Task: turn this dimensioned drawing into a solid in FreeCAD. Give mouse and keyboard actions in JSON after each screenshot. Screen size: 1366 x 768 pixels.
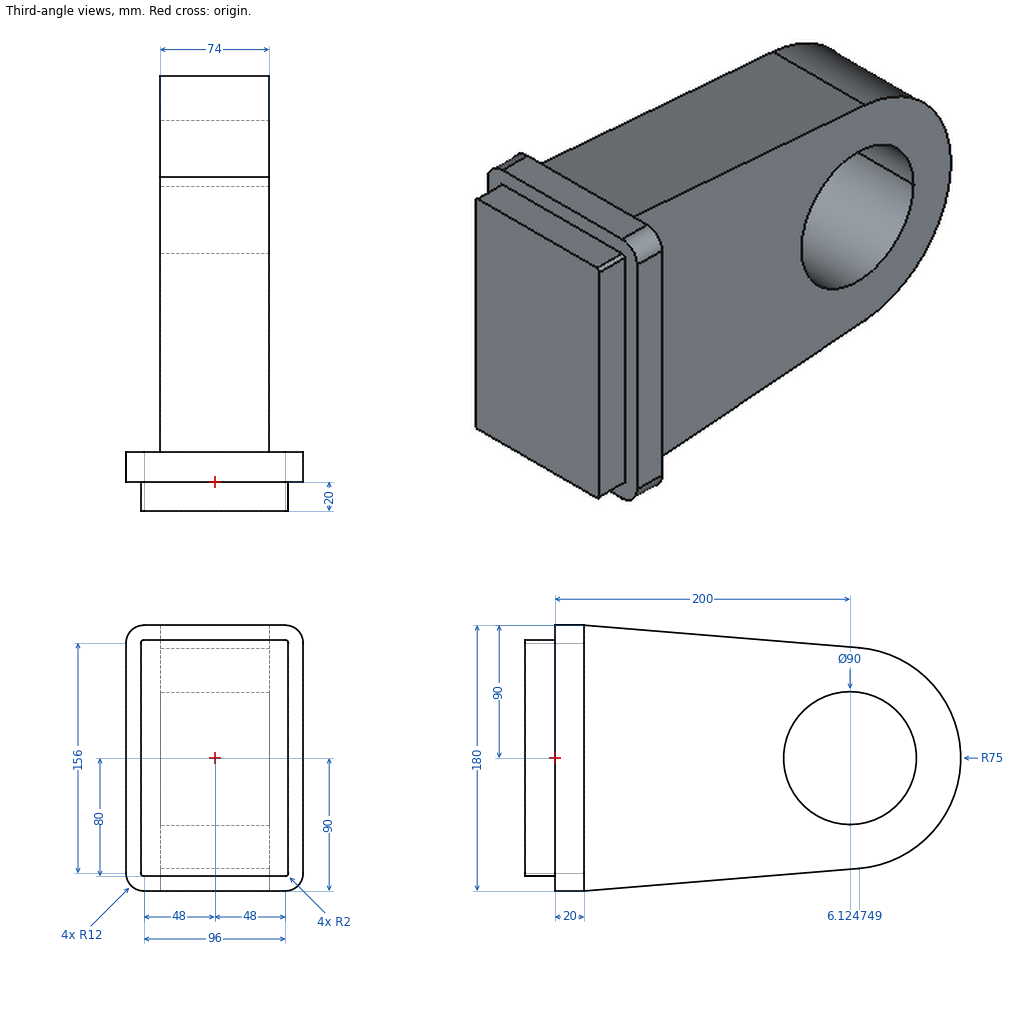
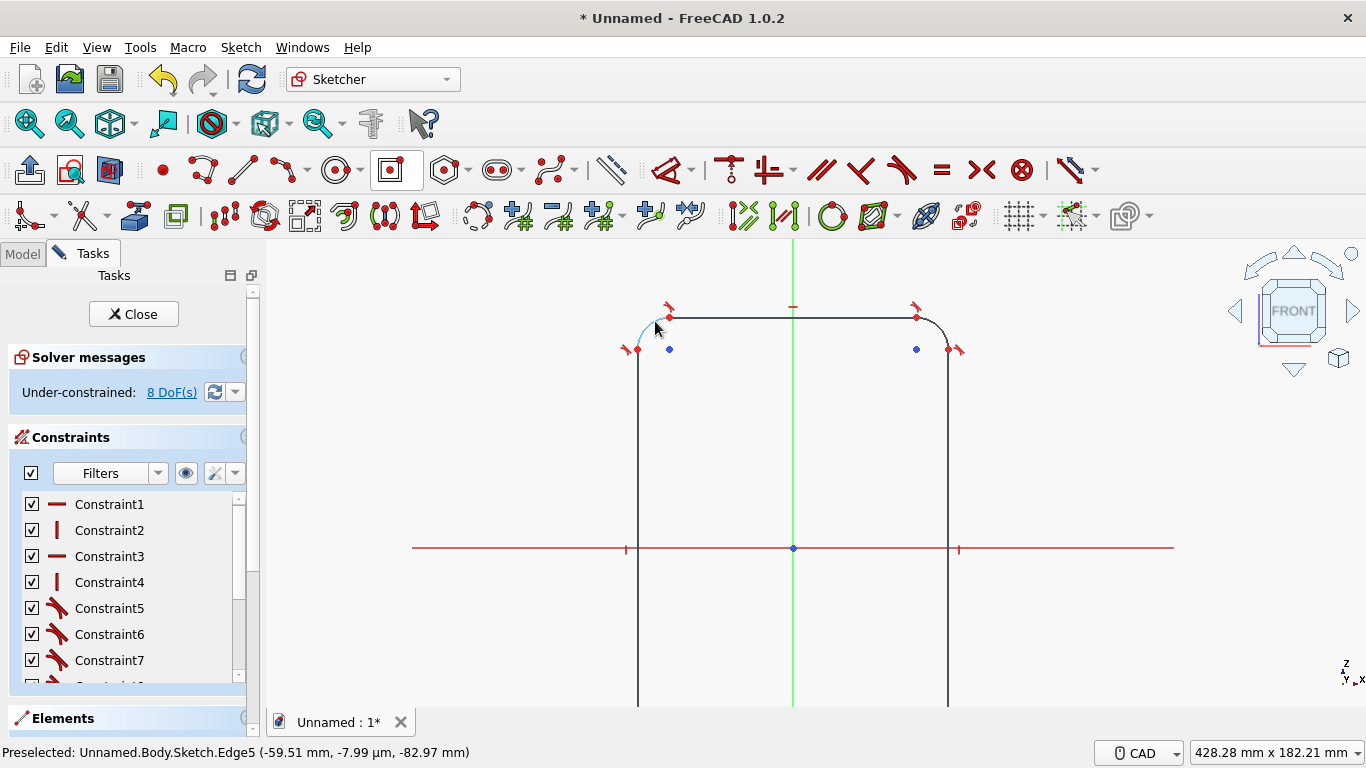
{"action": "left_click", "coordinate": [655, 321]}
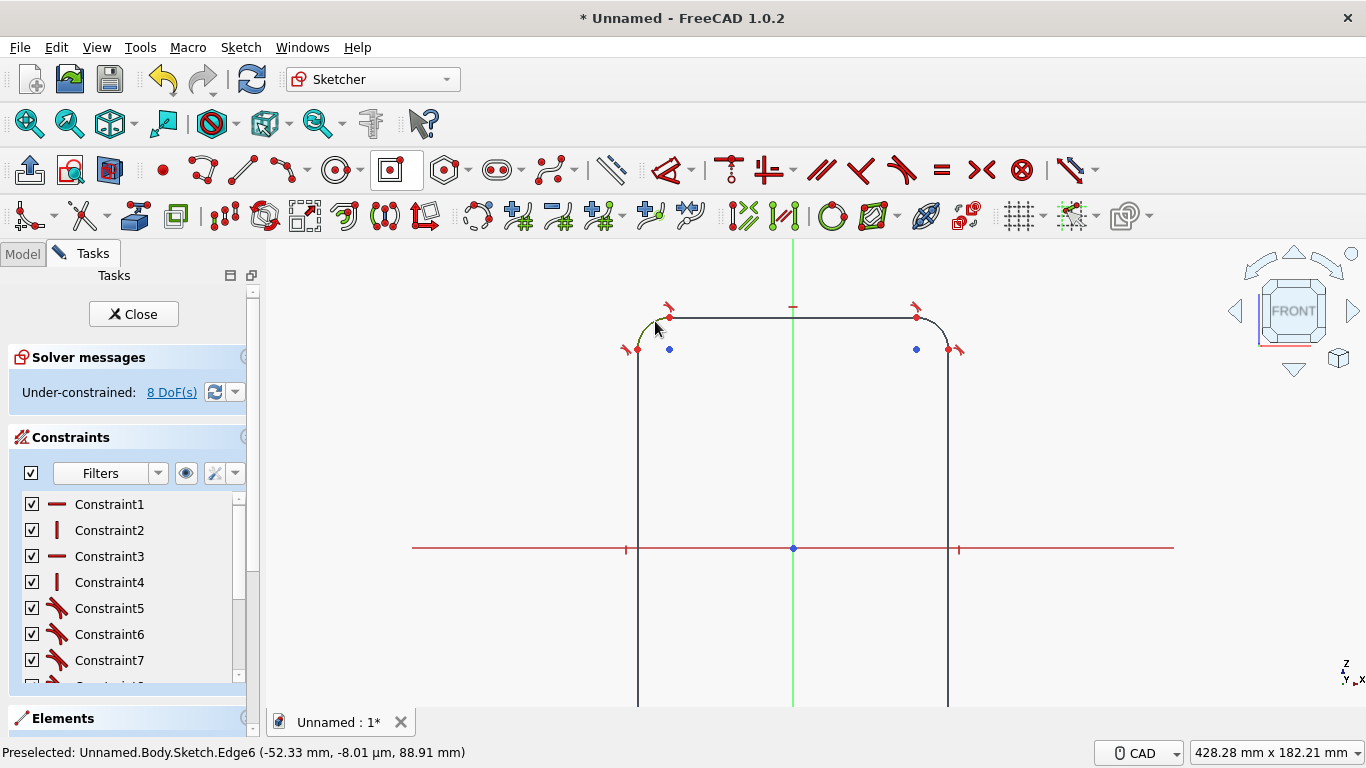
{"action": "left_click", "coordinate": [945, 335]}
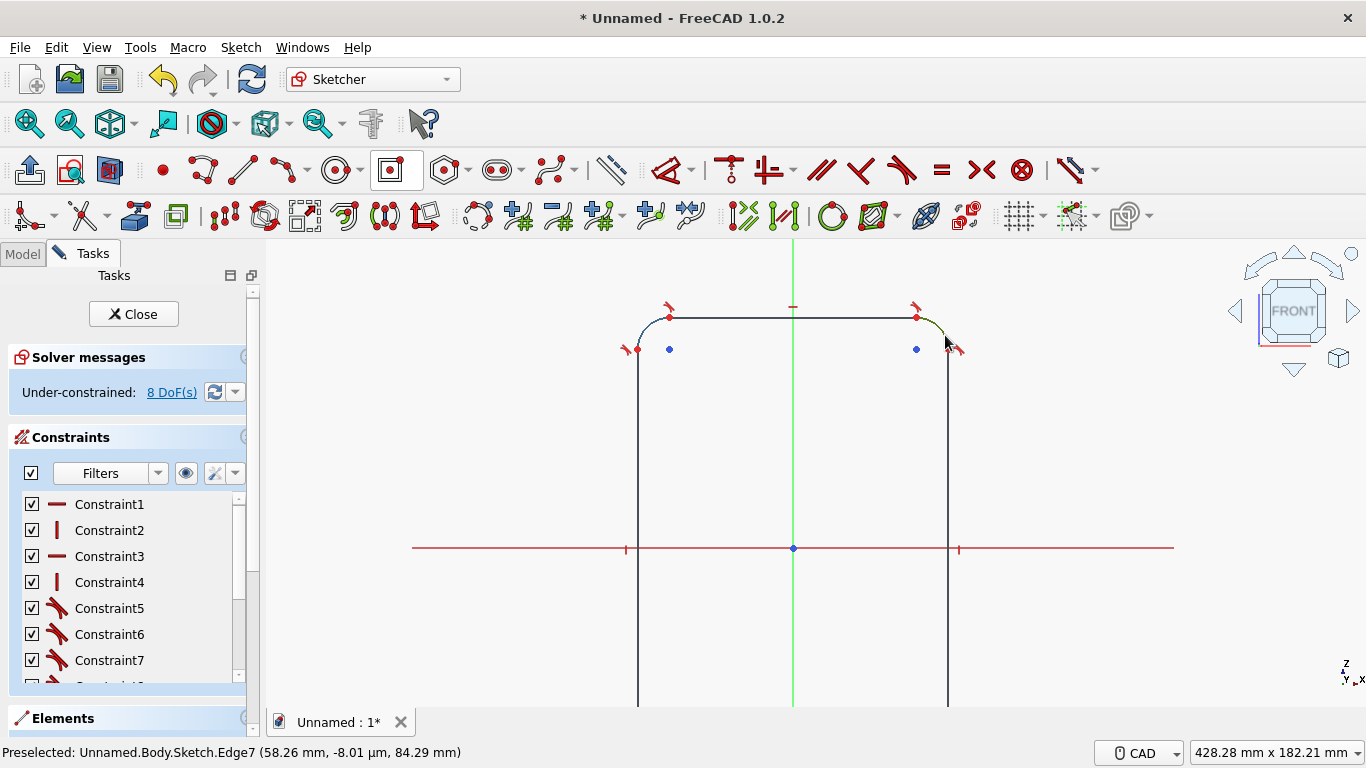
{"action": "scroll", "coordinate": [655, 320], "scroll_direction": "down", "scroll_amount": 2}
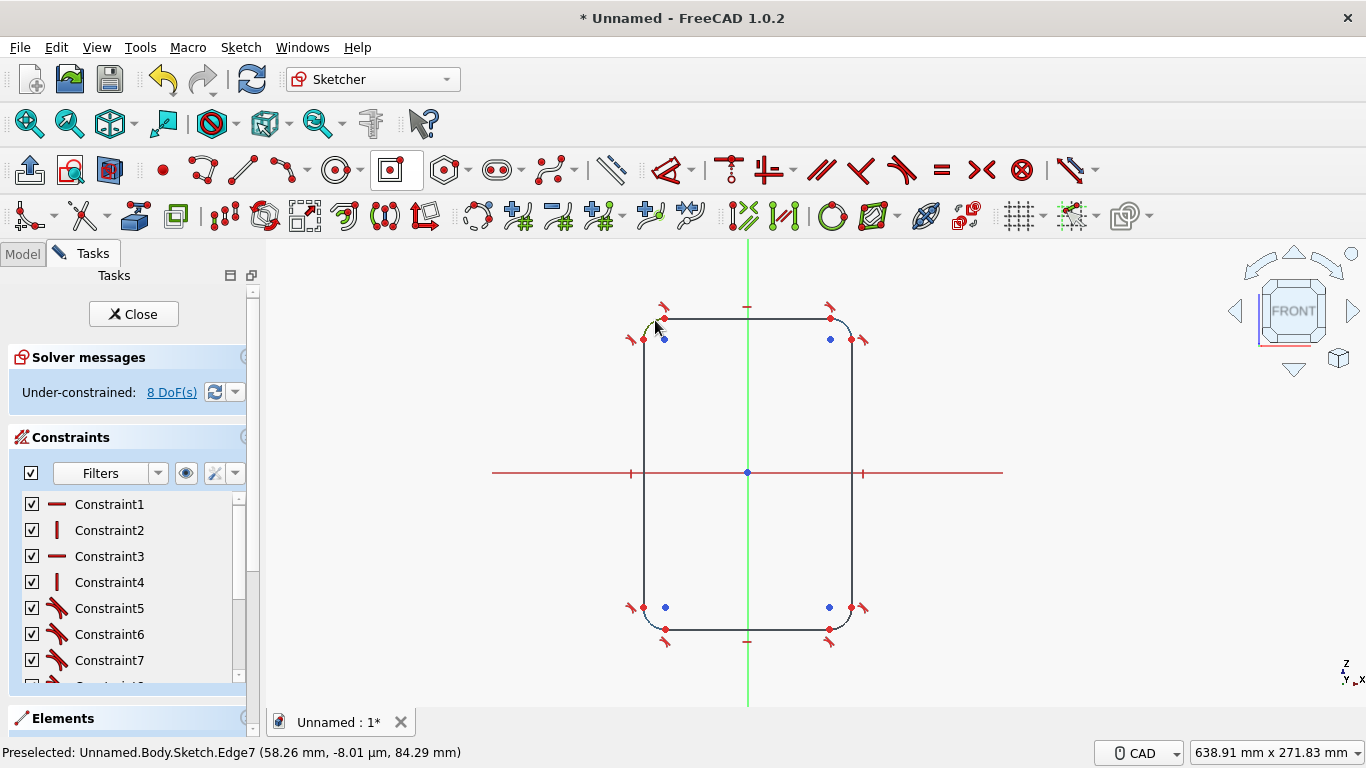
{"action": "scroll", "coordinate": [840, 627], "scroll_direction": "up", "scroll_amount": 2}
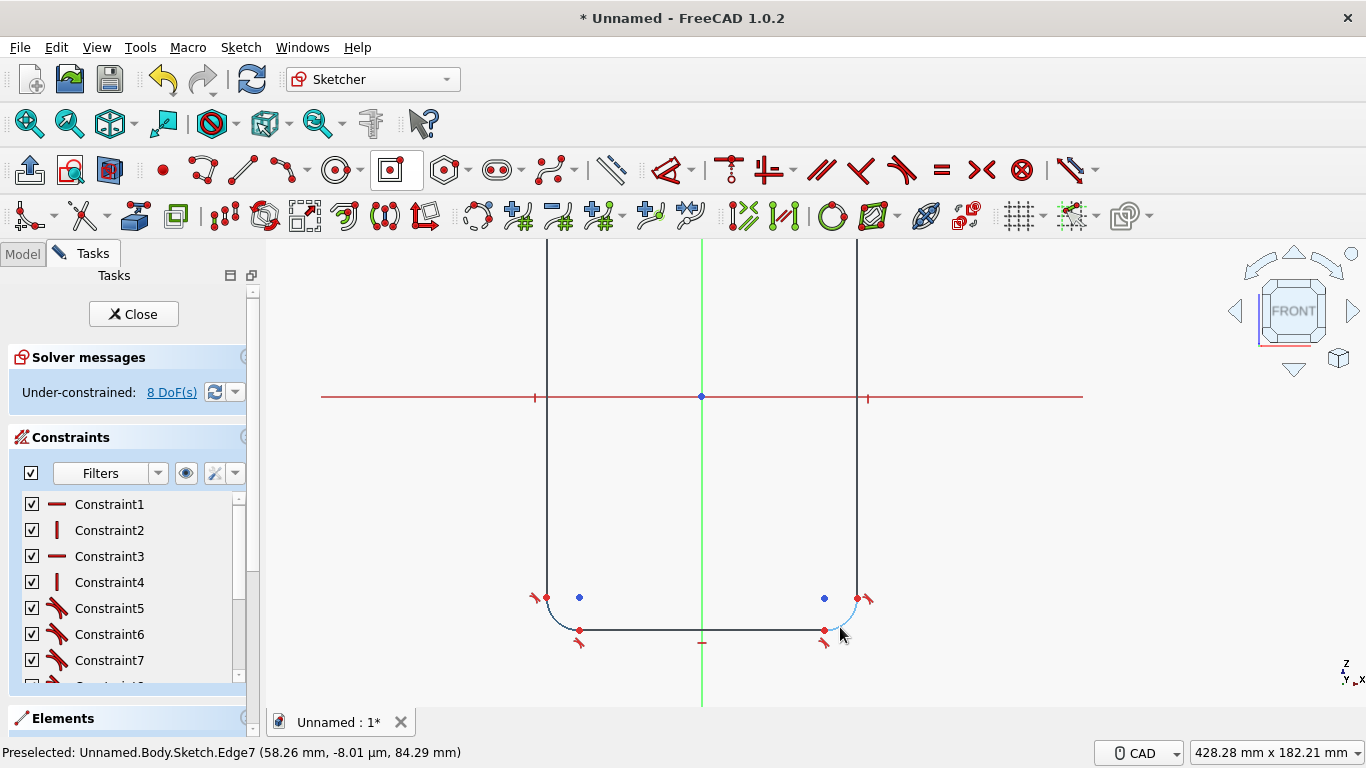
{"action": "left_click", "coordinate": [839, 627]}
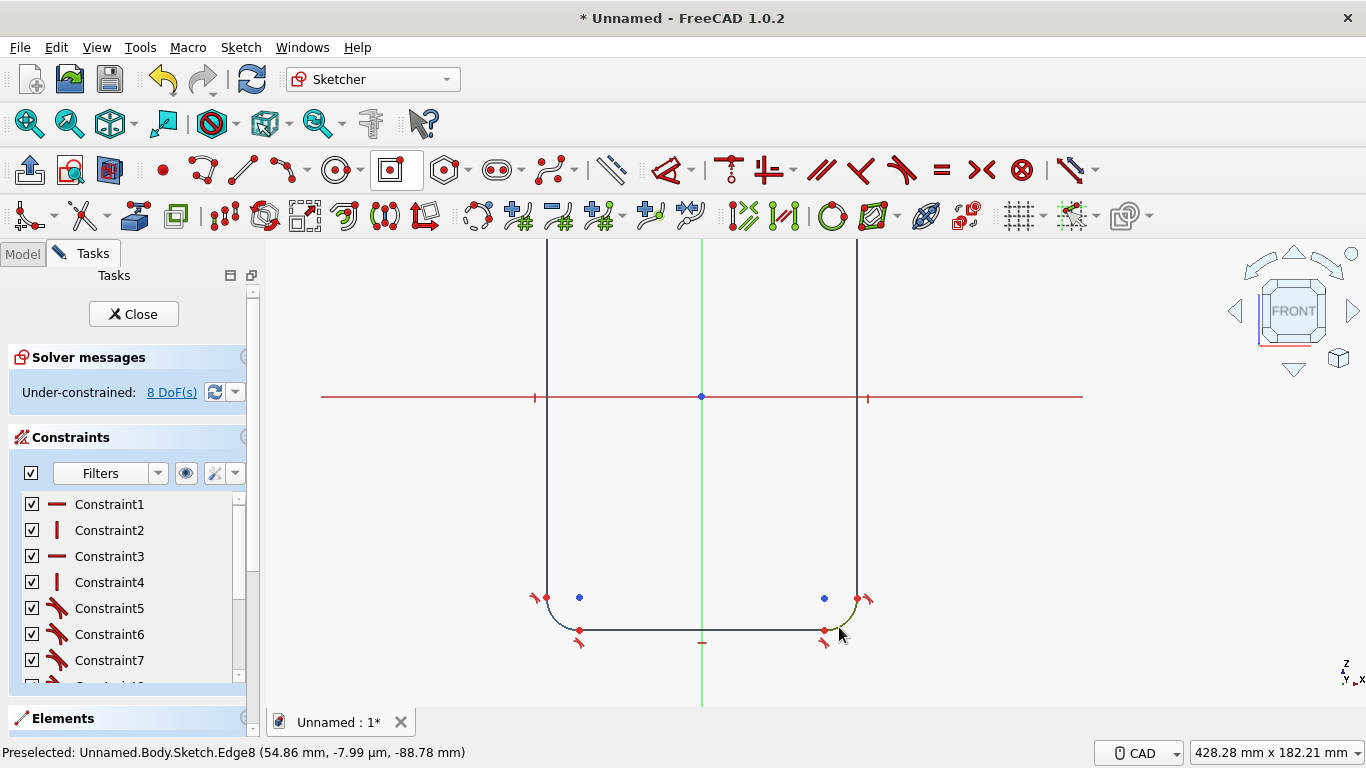
{"action": "key", "text": "e"}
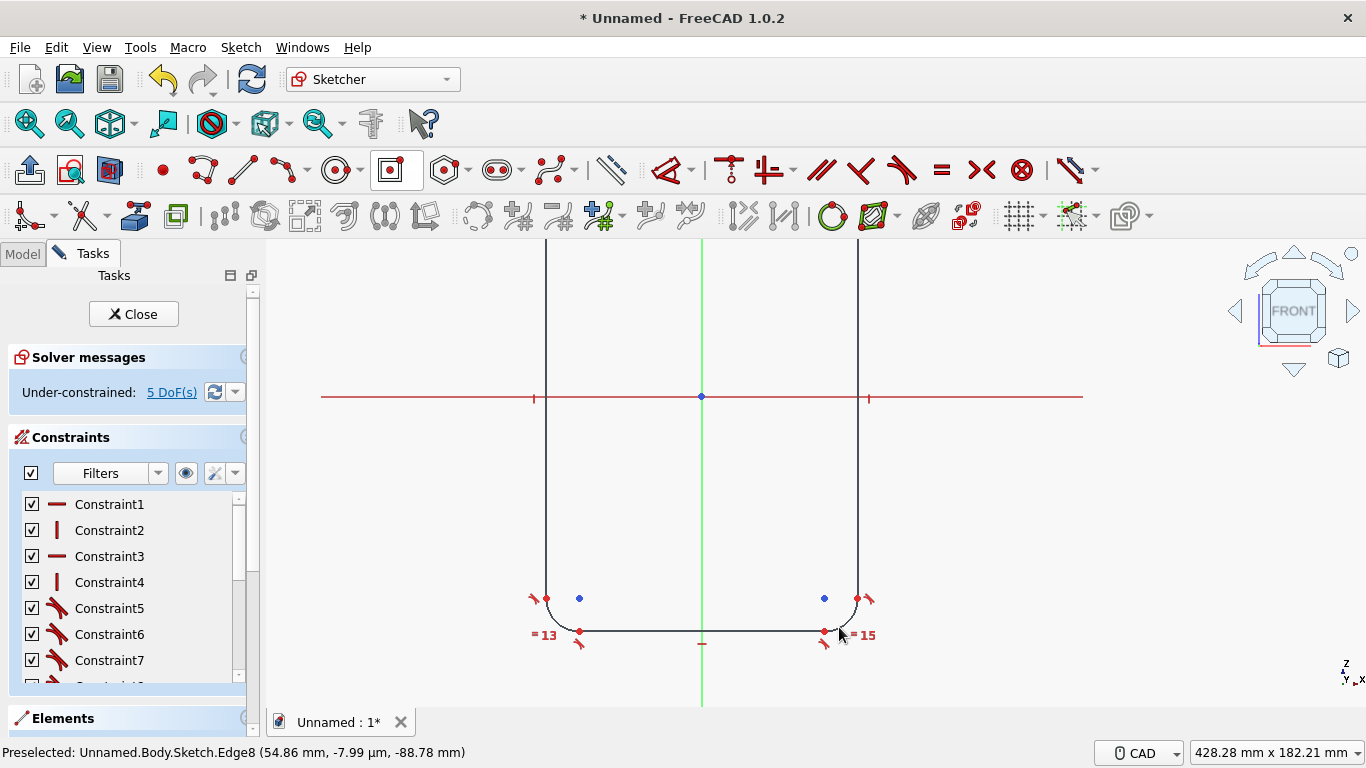
{"action": "key", "text": "d"}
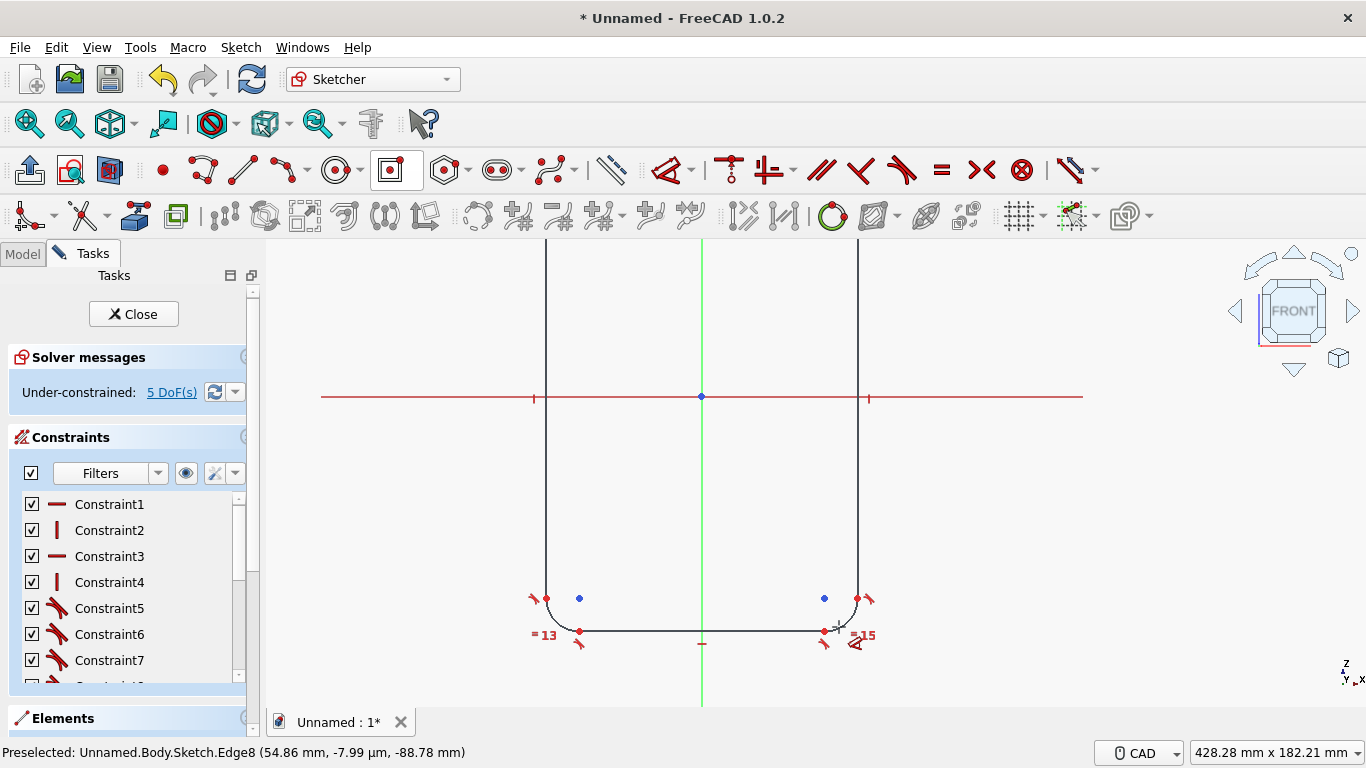
{"action": "scroll", "coordinate": [550, 613], "scroll_direction": "up", "scroll_amount": 2}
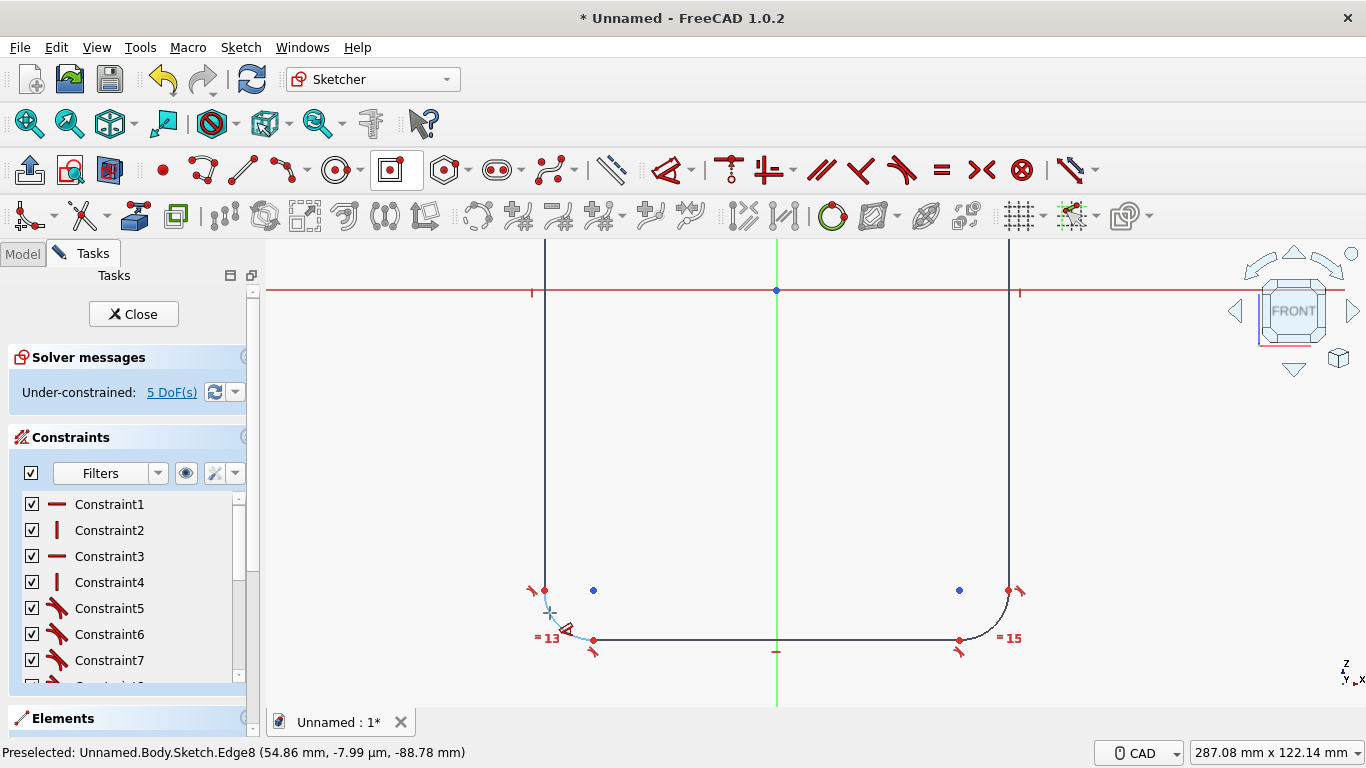
{"action": "left_click", "coordinate": [550, 613]}
{"action": "left_click", "coordinate": [521, 627]}